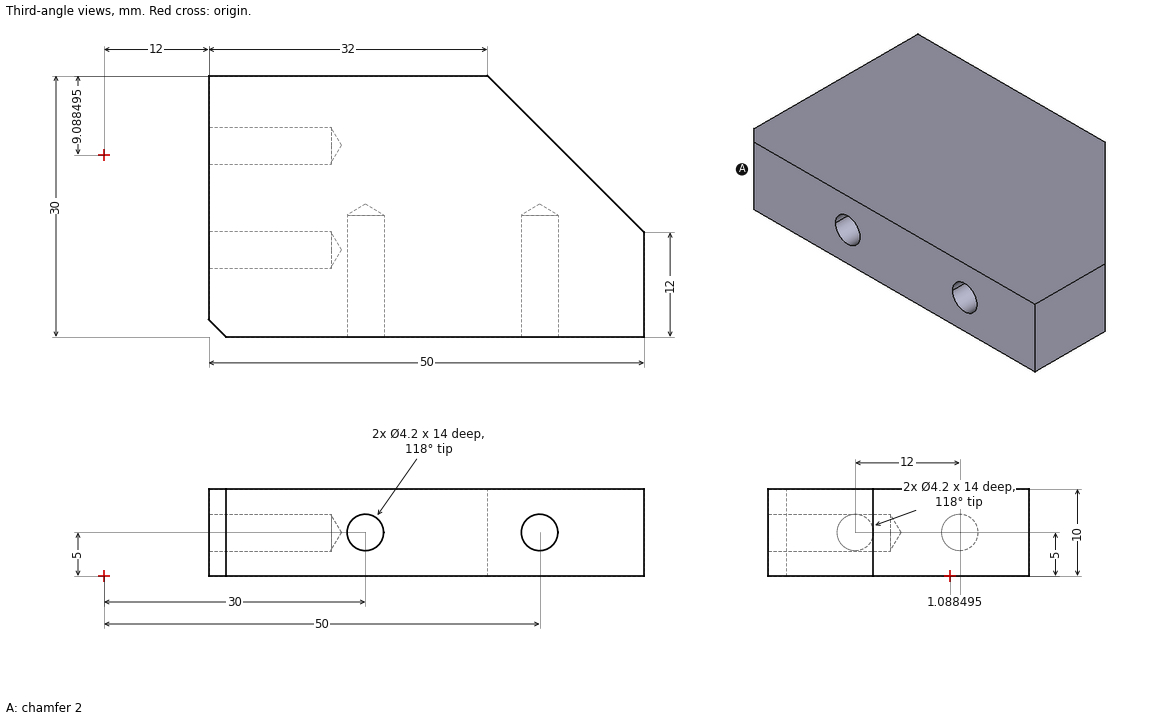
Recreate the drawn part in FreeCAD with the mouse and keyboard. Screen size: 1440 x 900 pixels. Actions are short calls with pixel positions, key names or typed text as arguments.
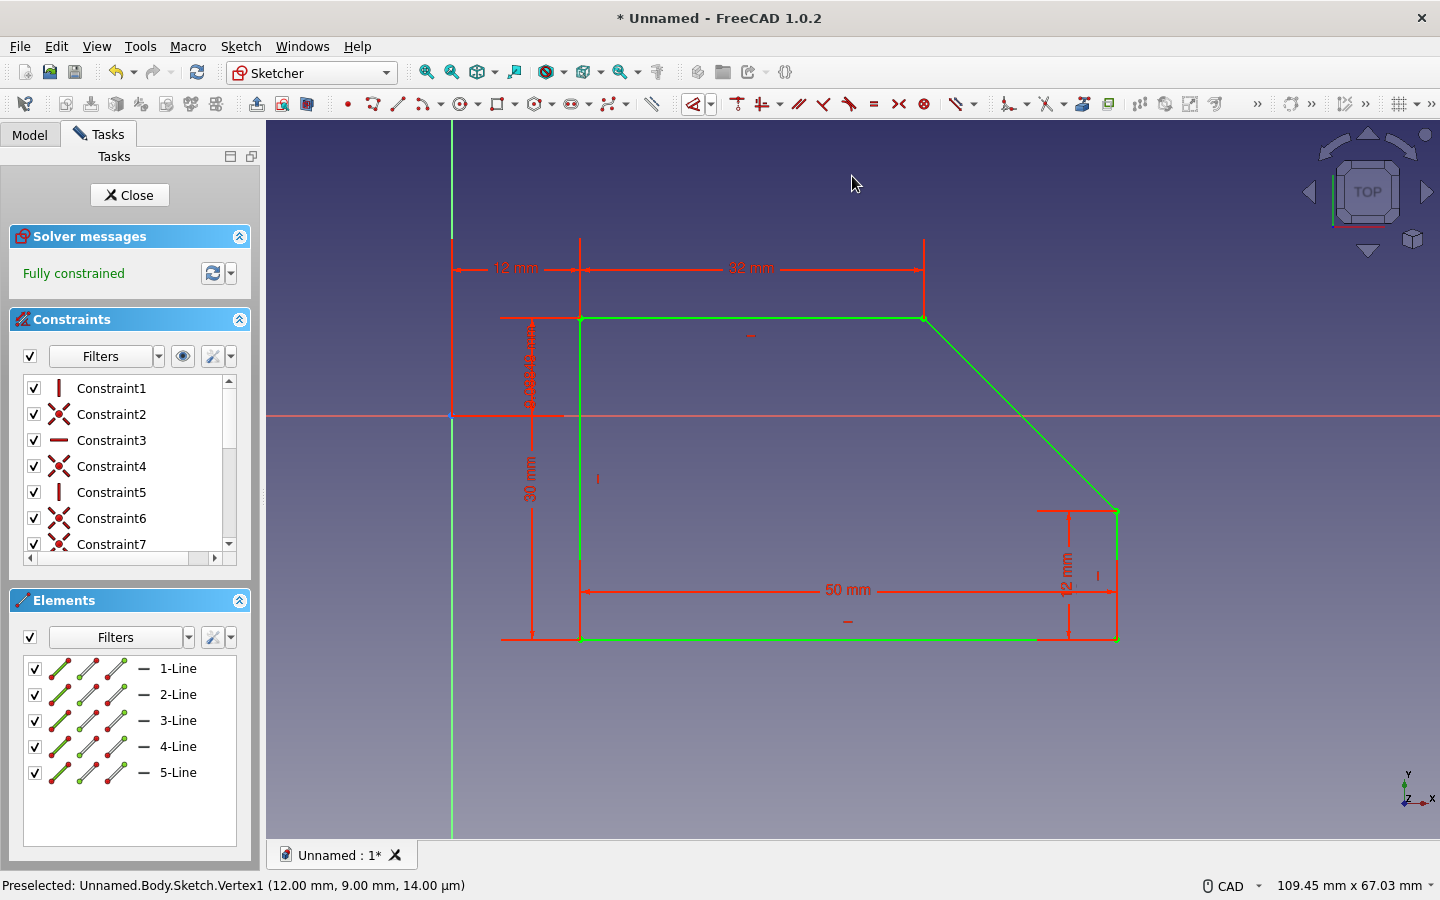
click(130, 195)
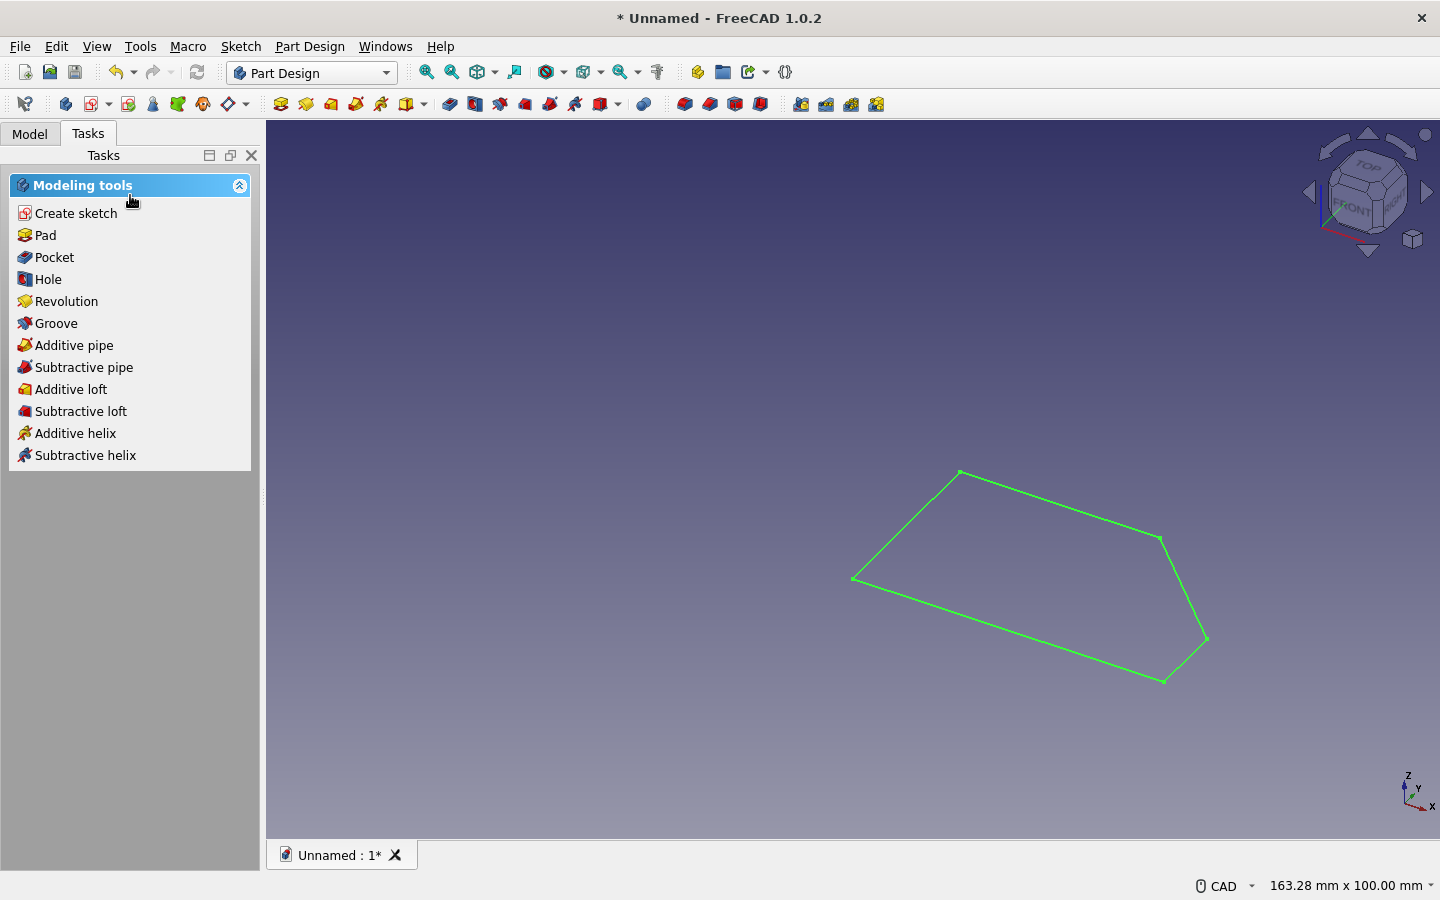
click(281, 104)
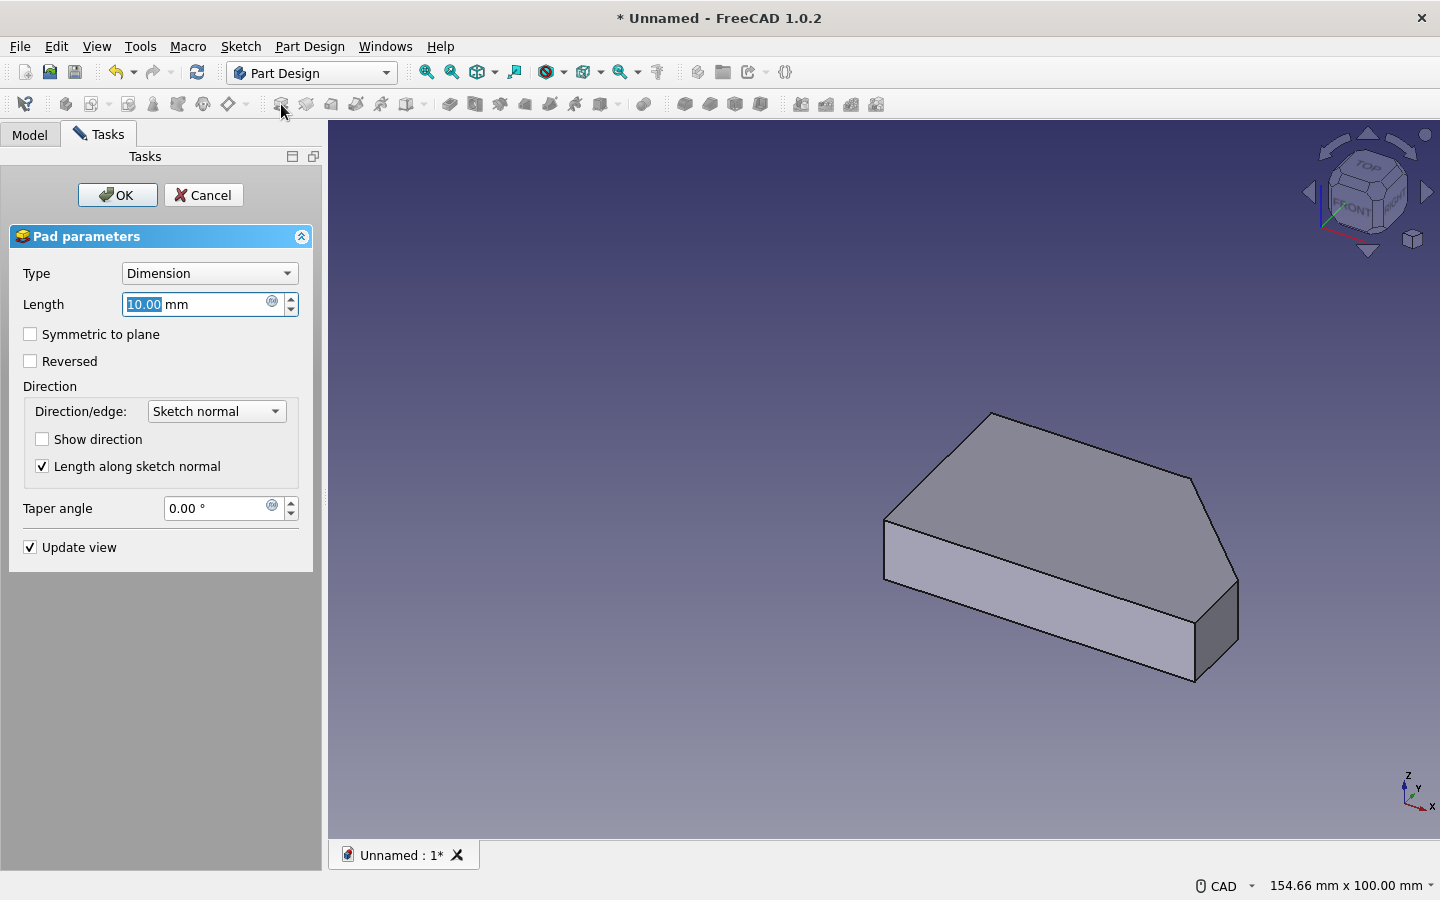
text(10)
key(Tab)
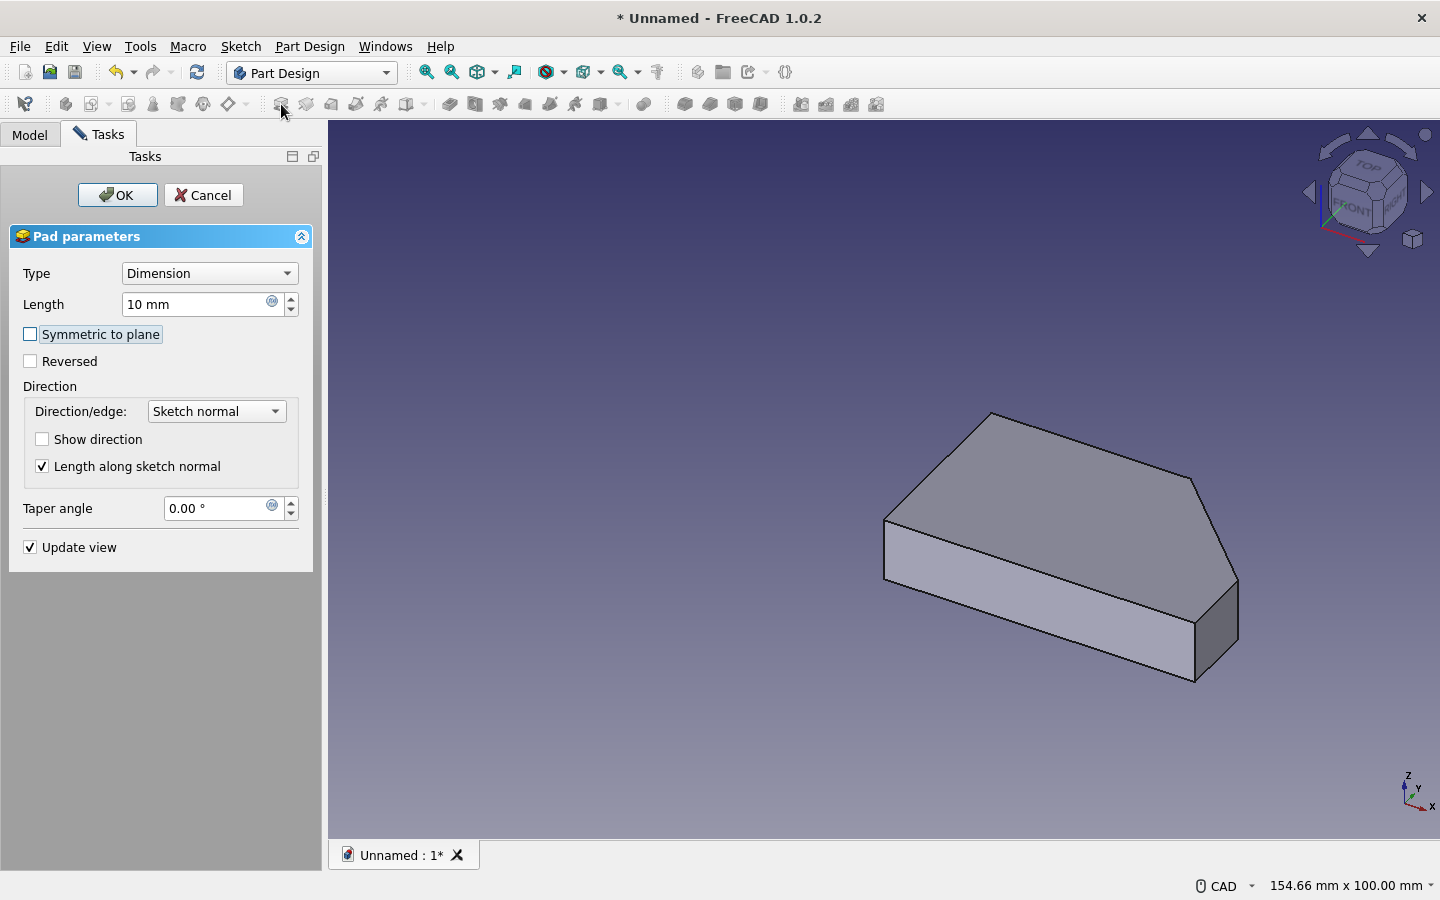
click(118, 195)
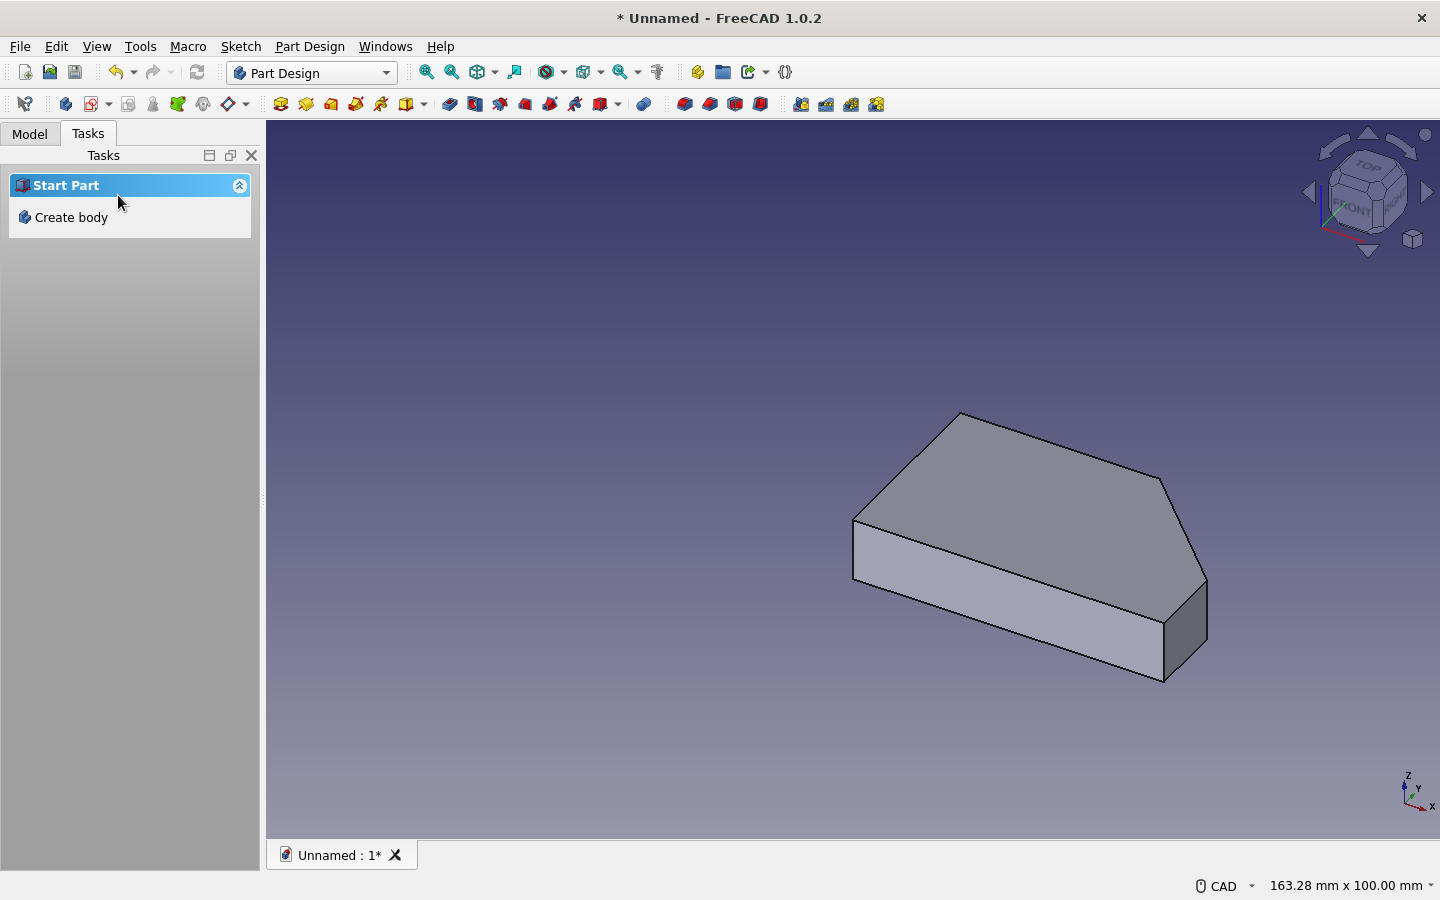
click(427, 72)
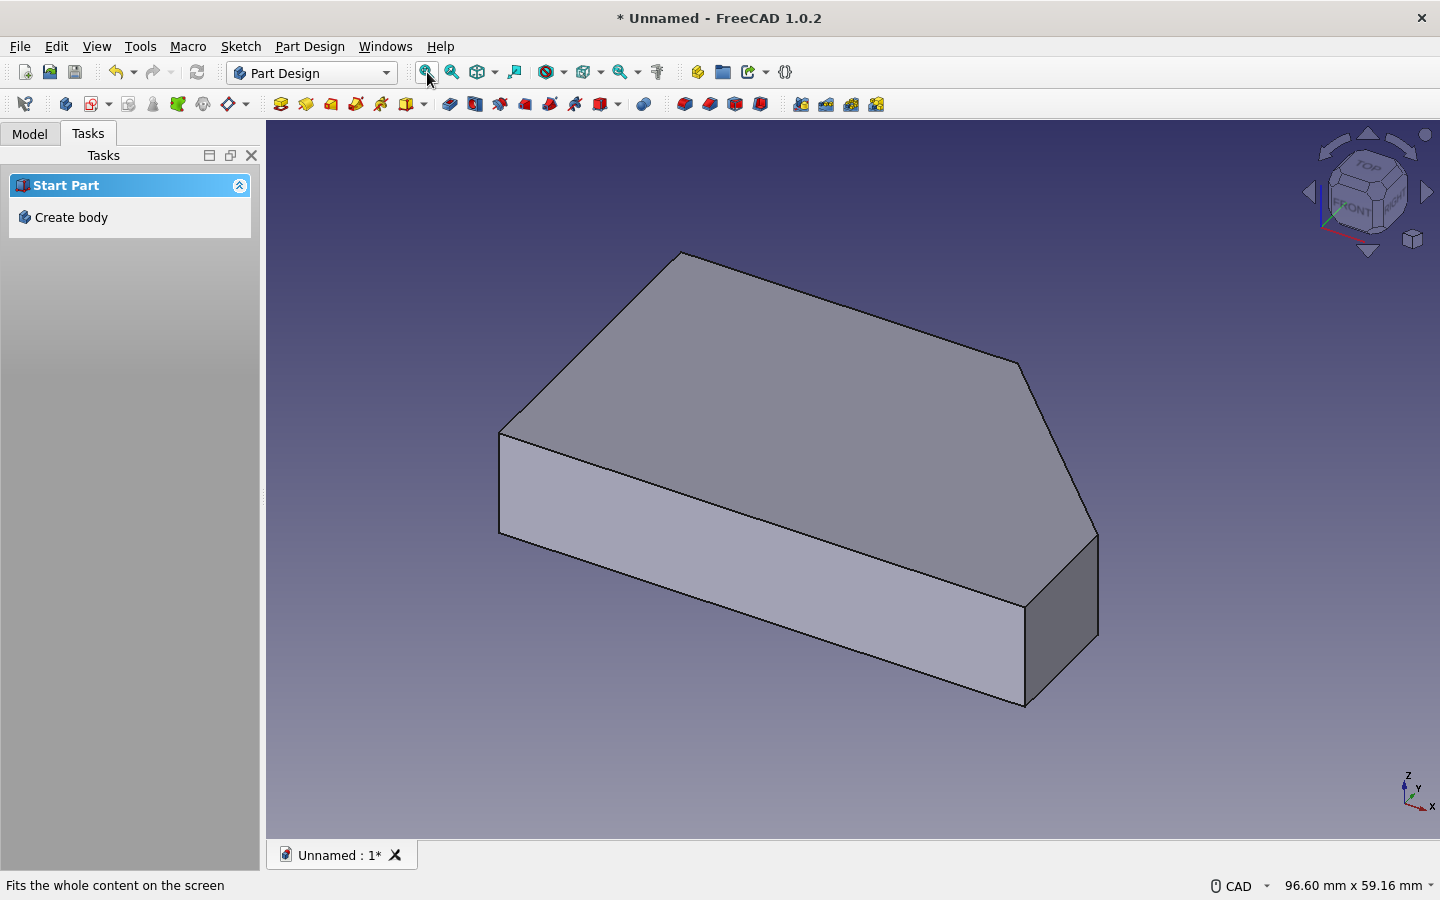
key(0)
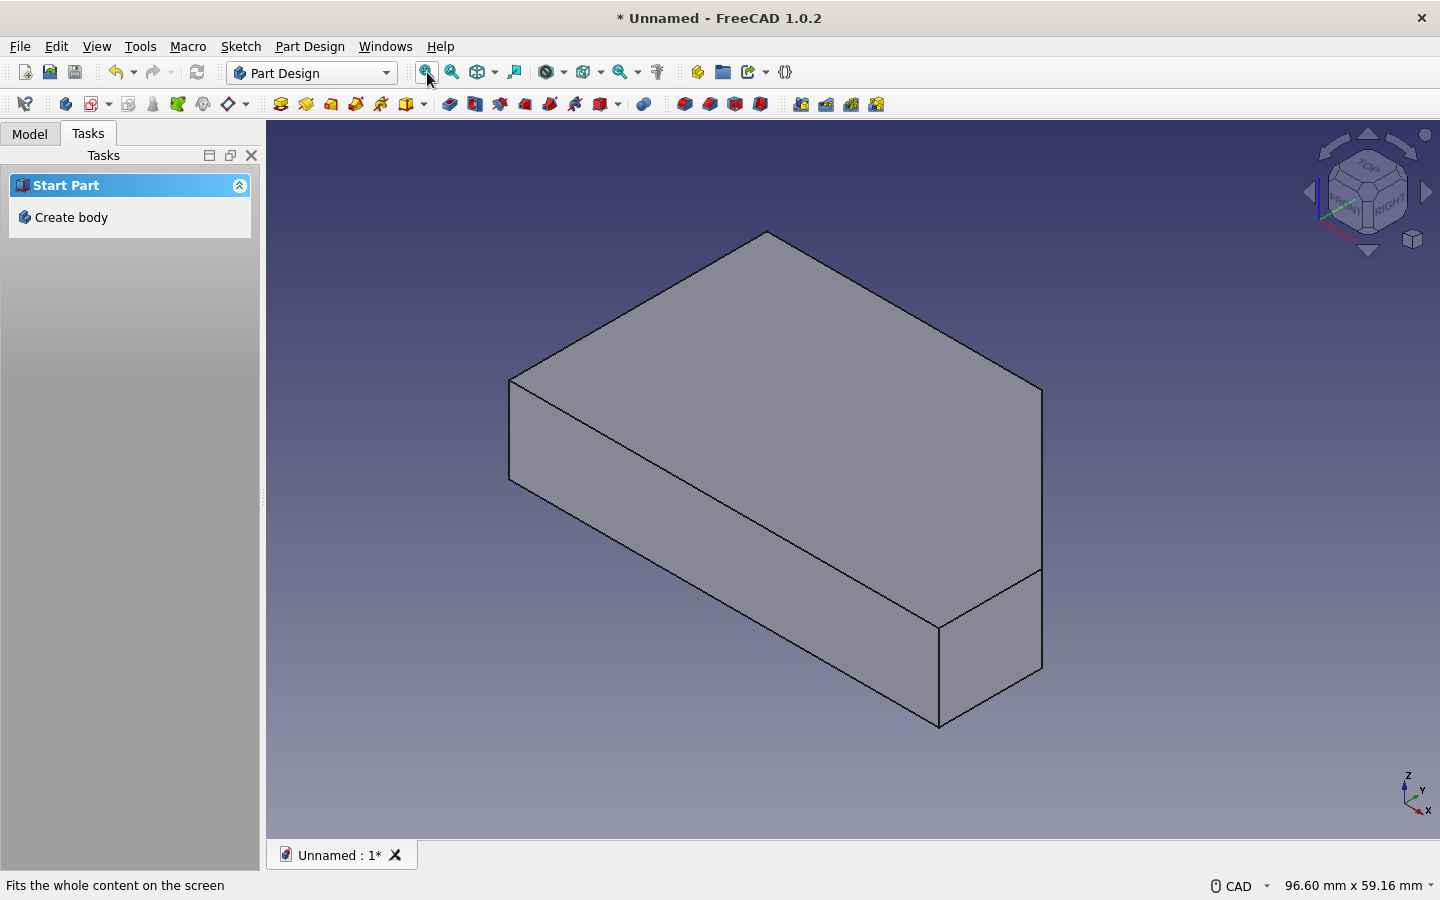
key(2)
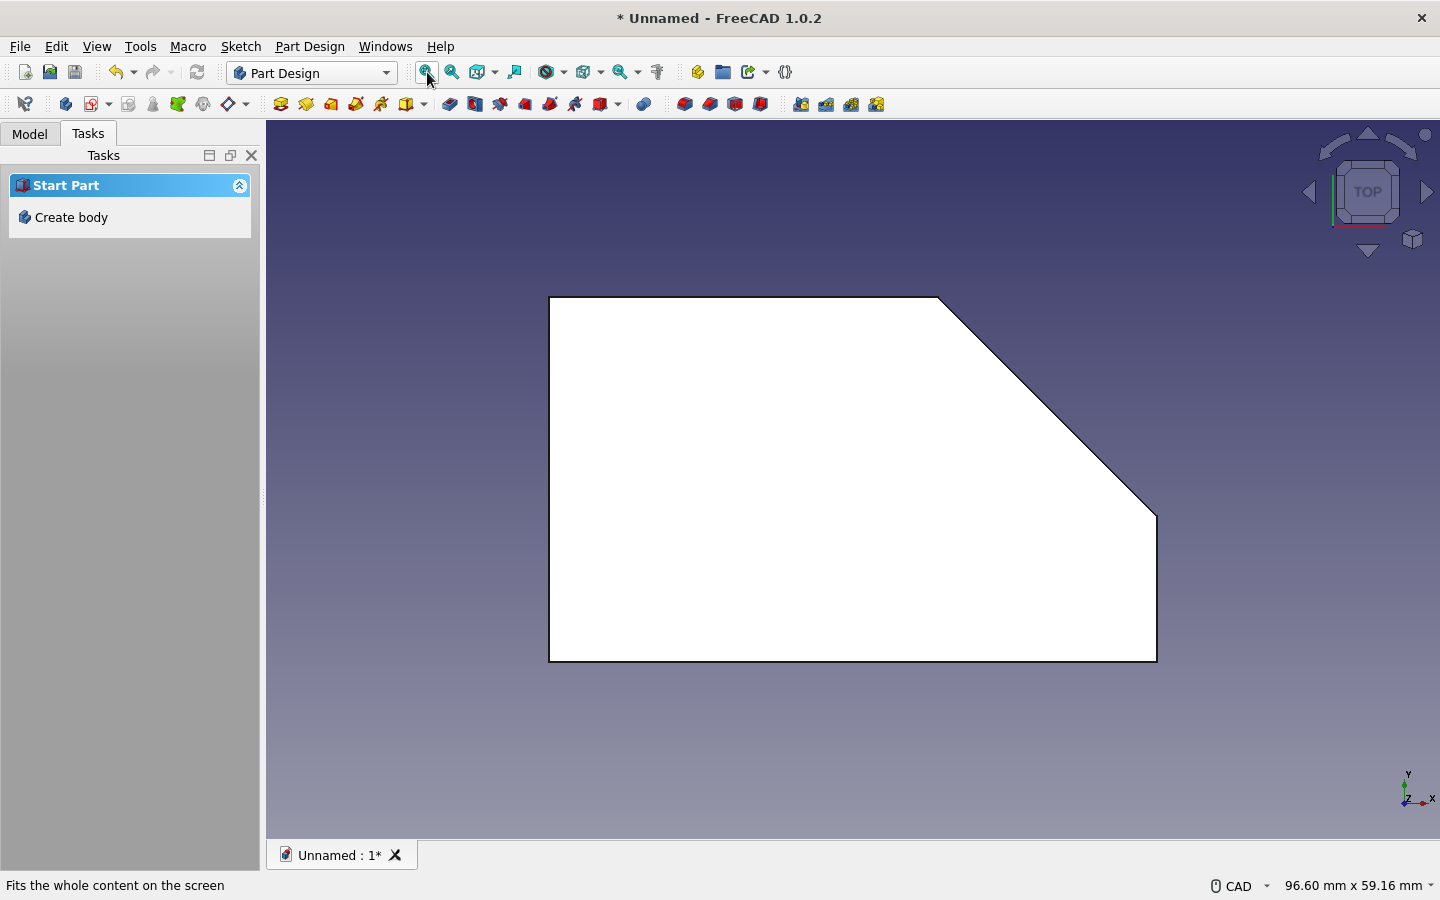
key(1)